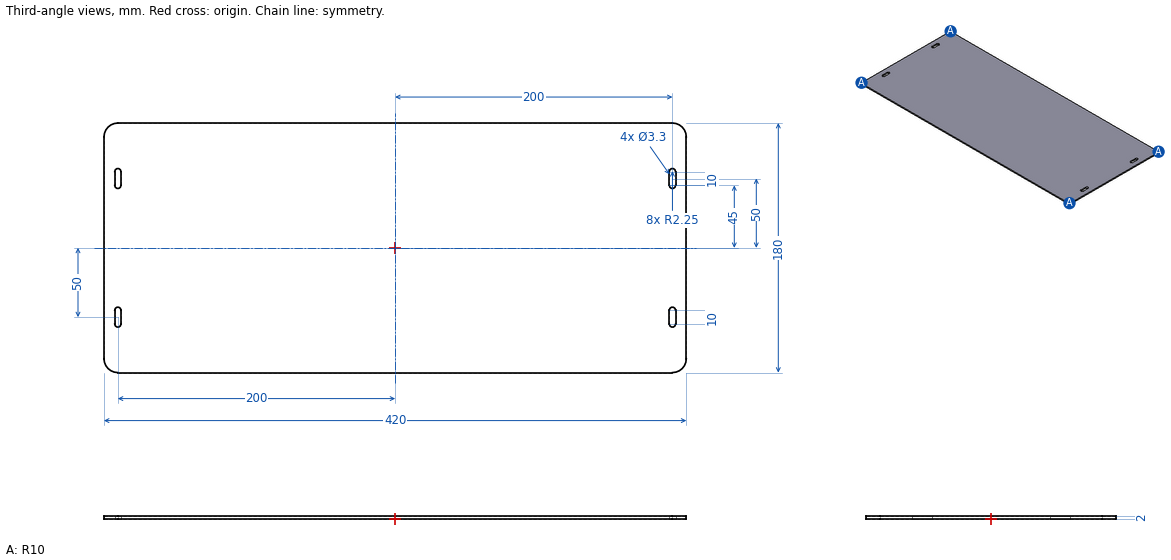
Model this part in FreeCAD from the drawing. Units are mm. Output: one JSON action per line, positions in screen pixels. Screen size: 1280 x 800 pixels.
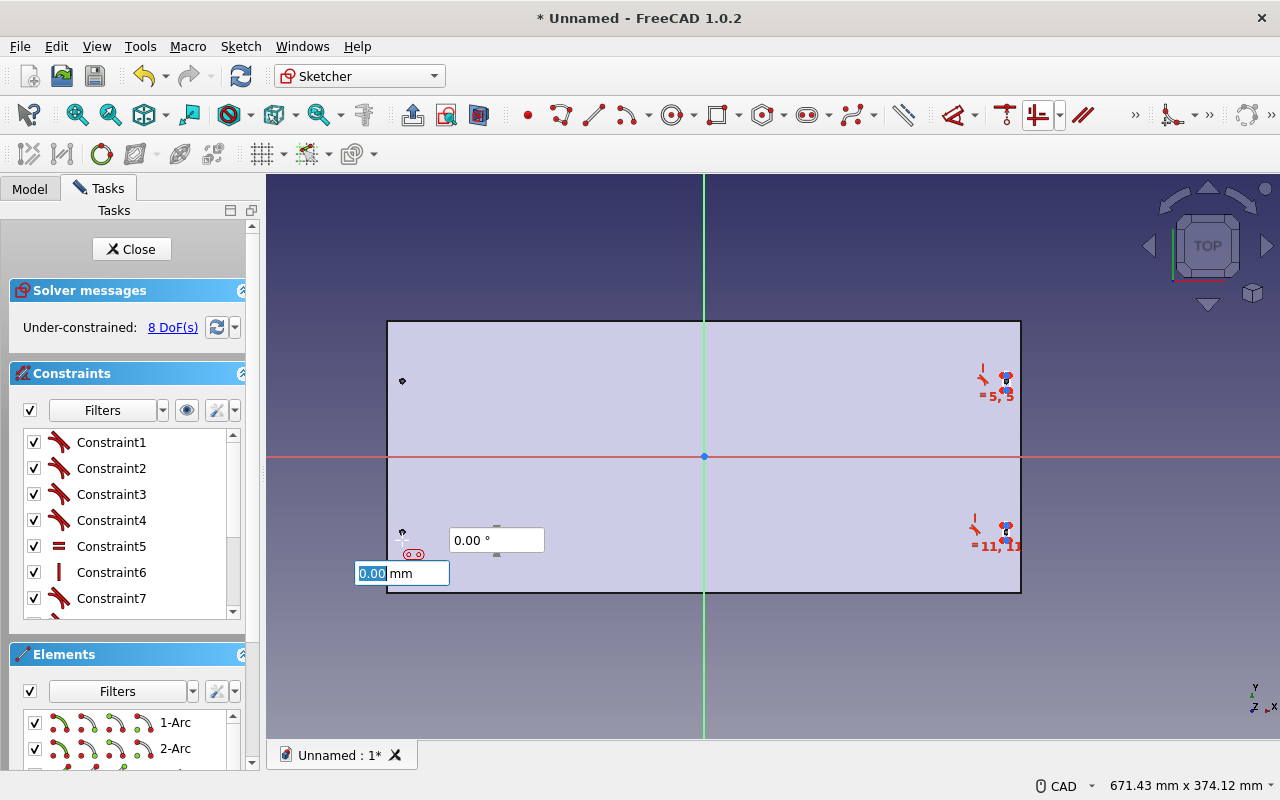
{"action": "left_click", "coordinate": [402, 525]}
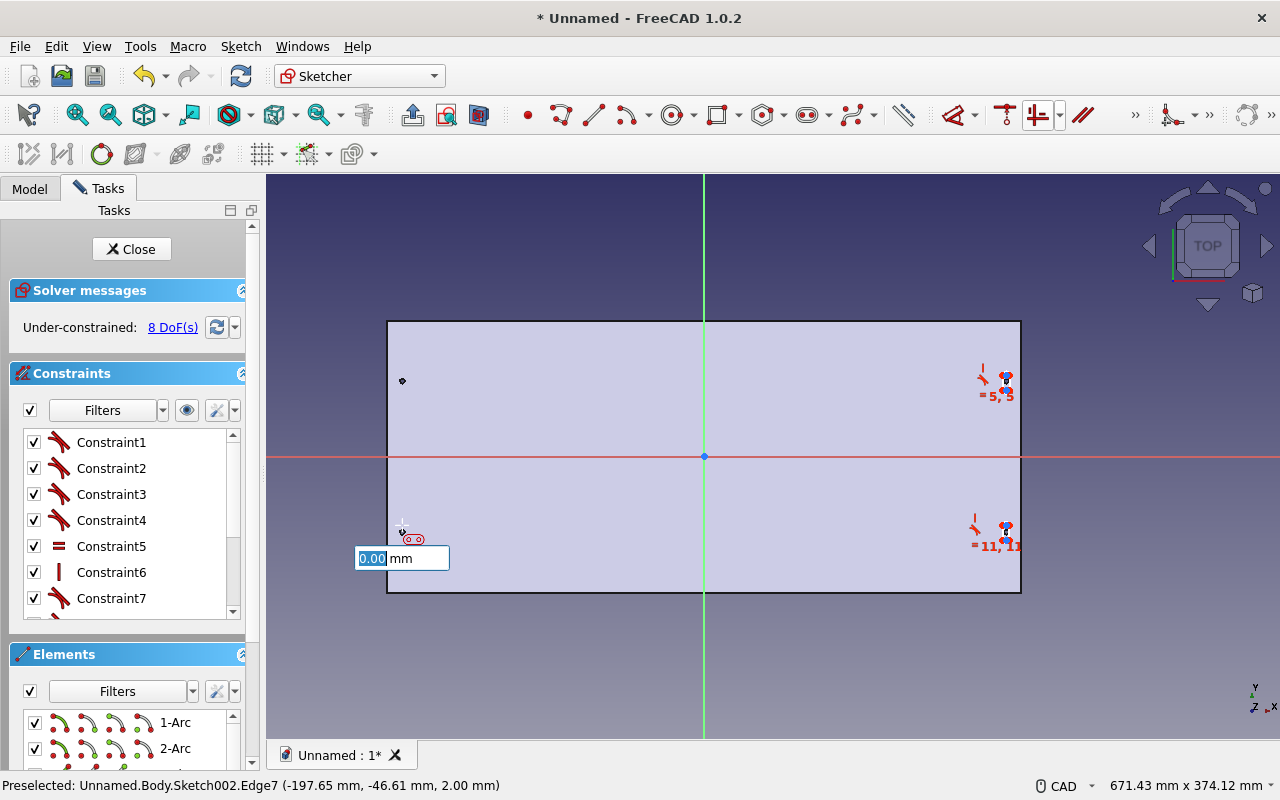
{"action": "scroll", "coordinate": [406, 532], "scroll_direction": "up", "scroll_amount": 8}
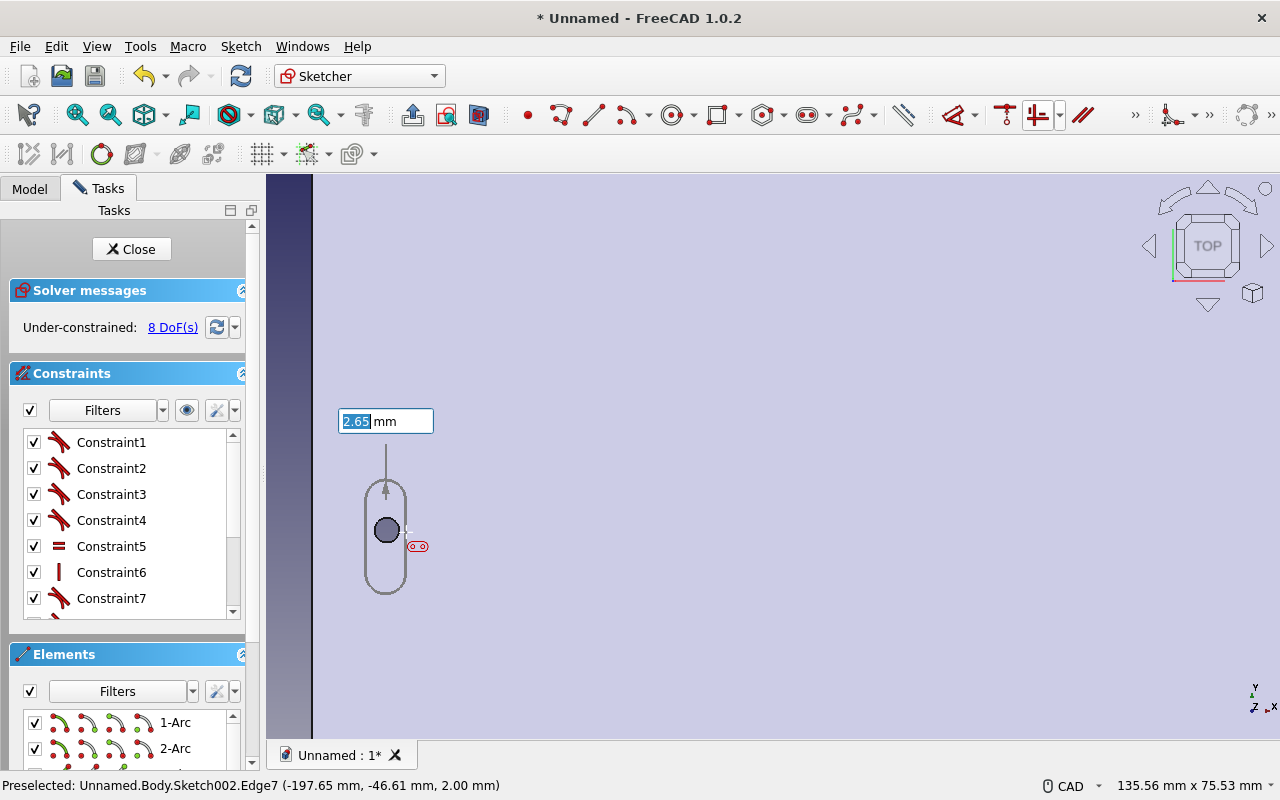
{"action": "left_click", "coordinate": [404, 530]}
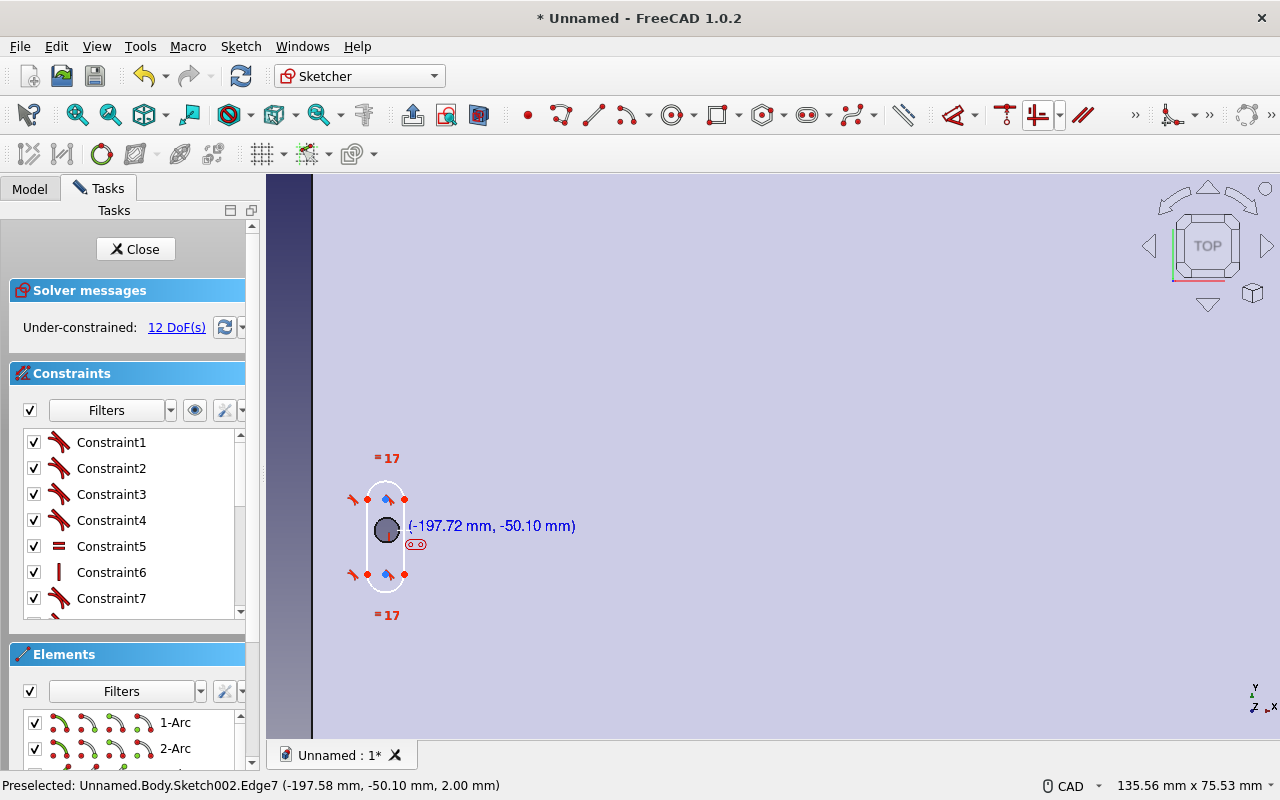
{"action": "scroll", "coordinate": [406, 532], "scroll_direction": "down", "scroll_amount": 8}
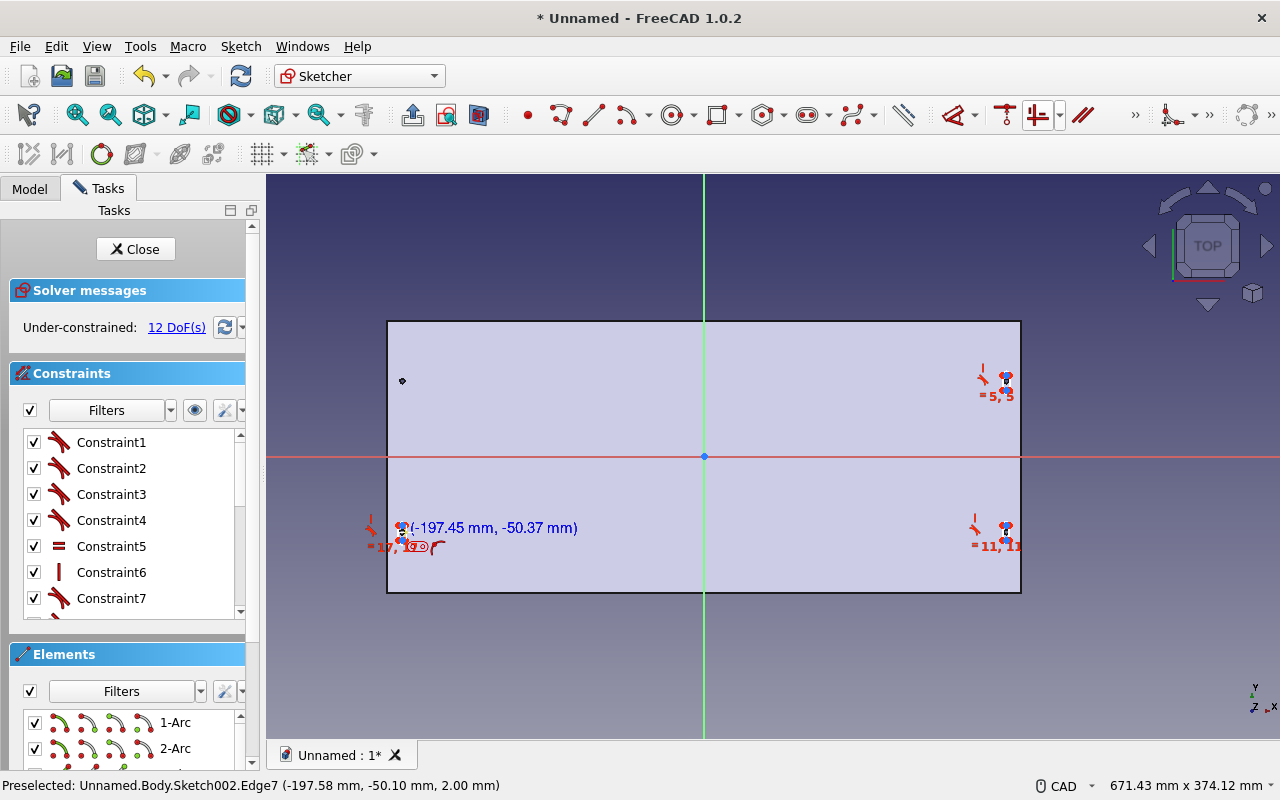
{"action": "scroll", "coordinate": [402, 389], "scroll_direction": "up", "scroll_amount": 10}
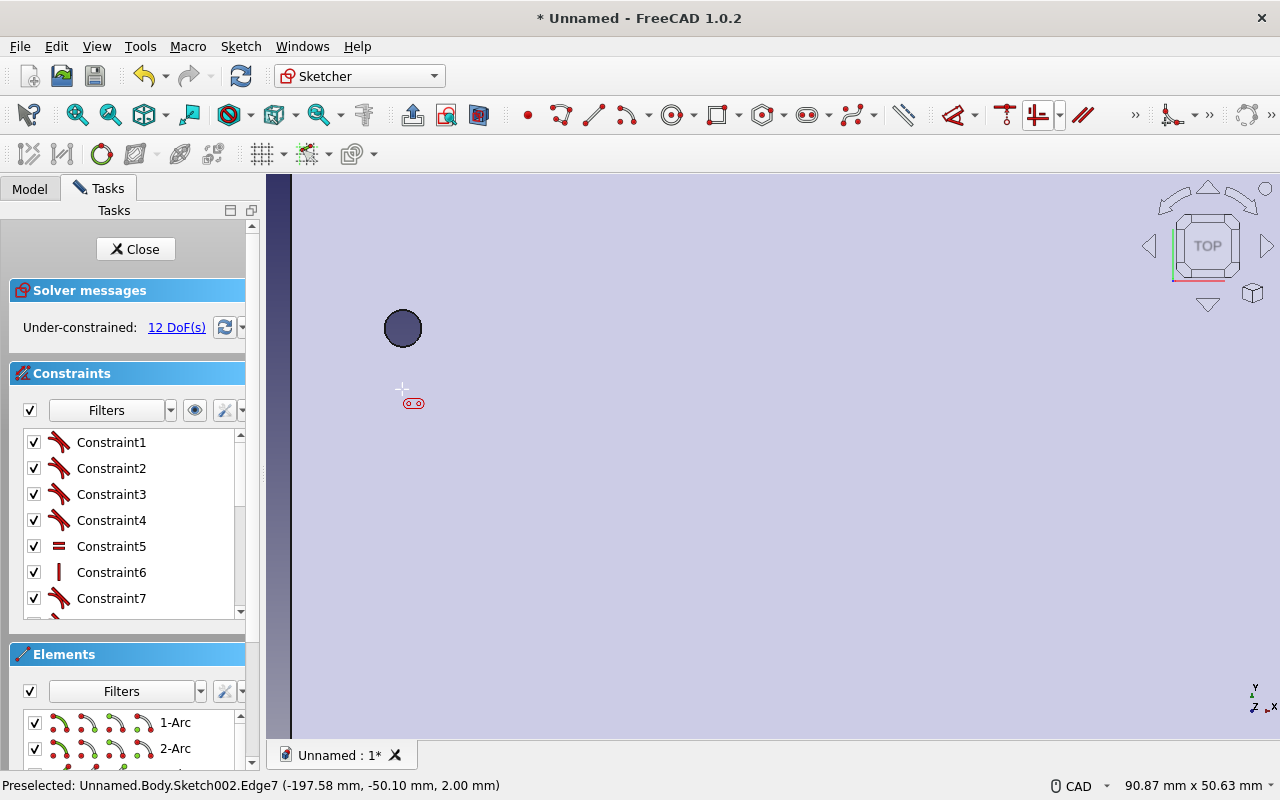
{"action": "scroll", "coordinate": [402, 389], "scroll_direction": "down", "scroll_amount": 10}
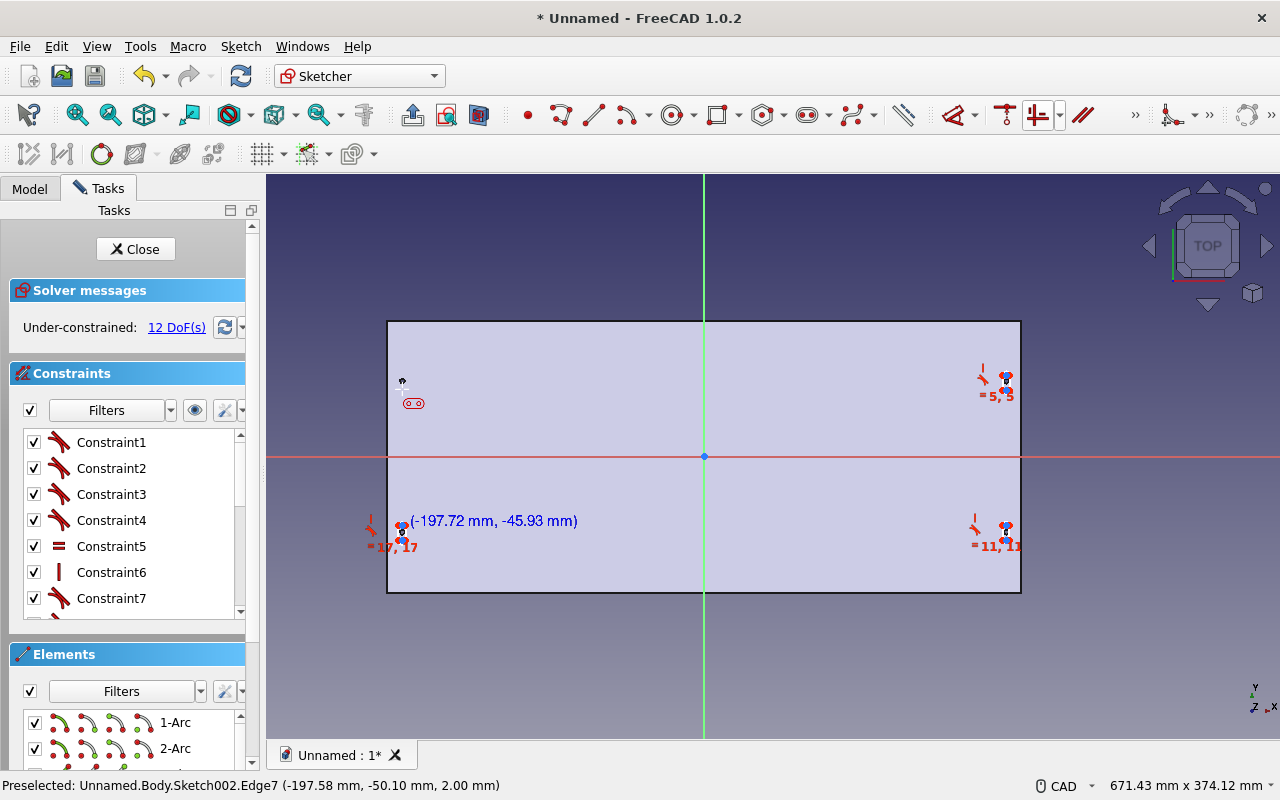
{"action": "left_click", "coordinate": [402, 389]}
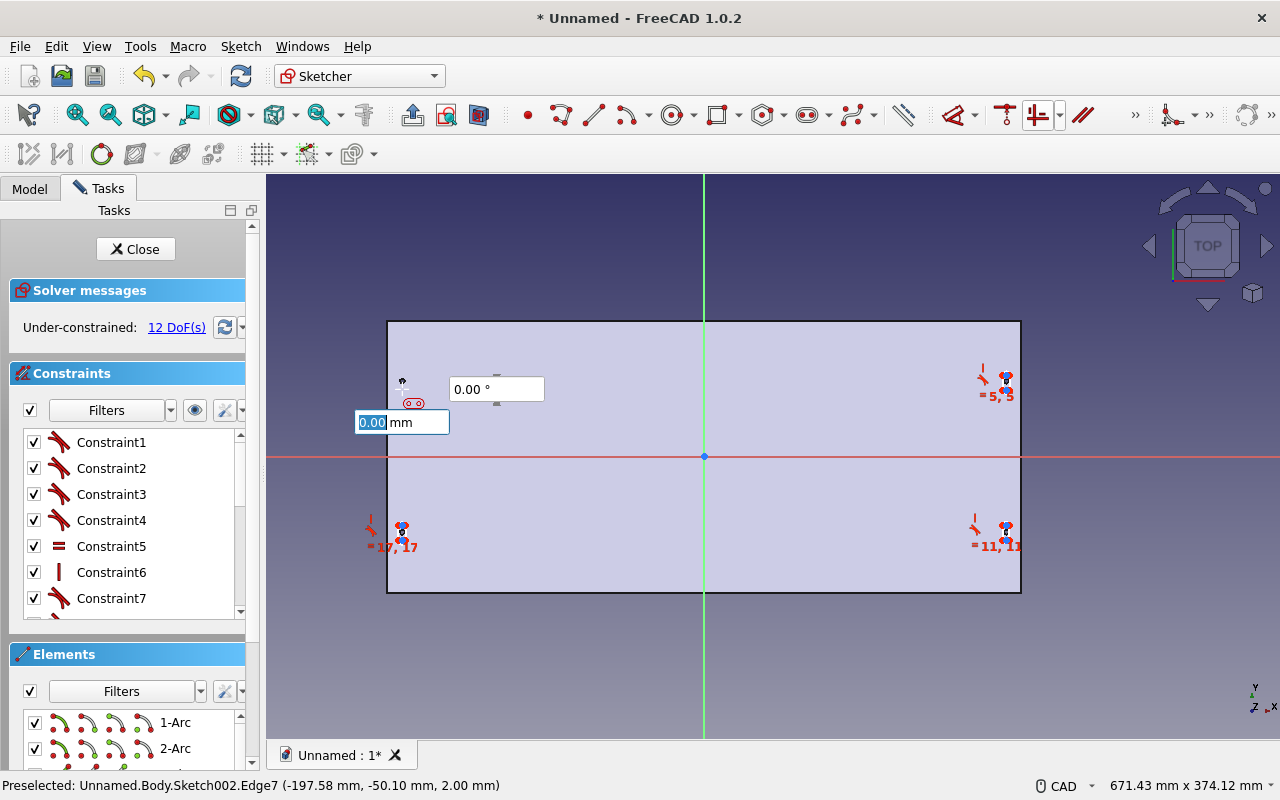
{"action": "left_click", "coordinate": [402, 374]}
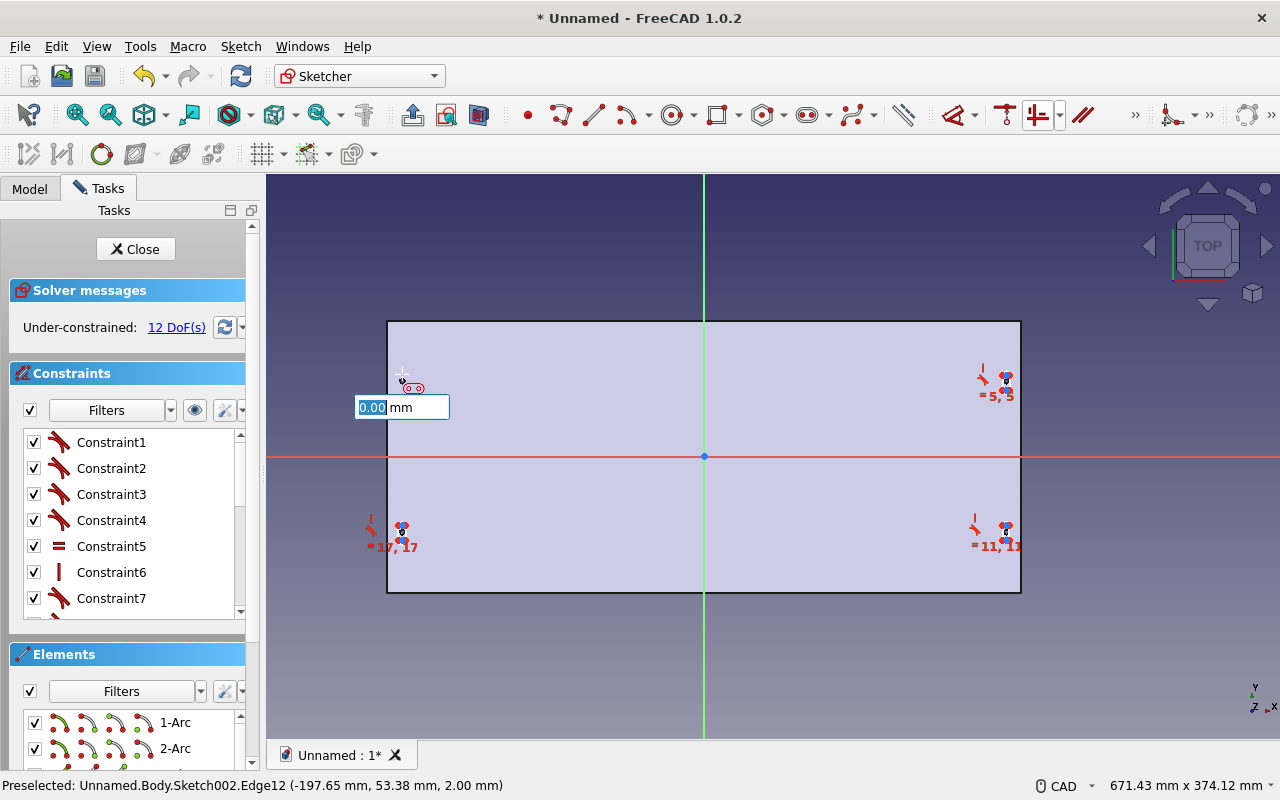
{"action": "scroll", "coordinate": [399, 381], "scroll_direction": "up", "scroll_amount": 8}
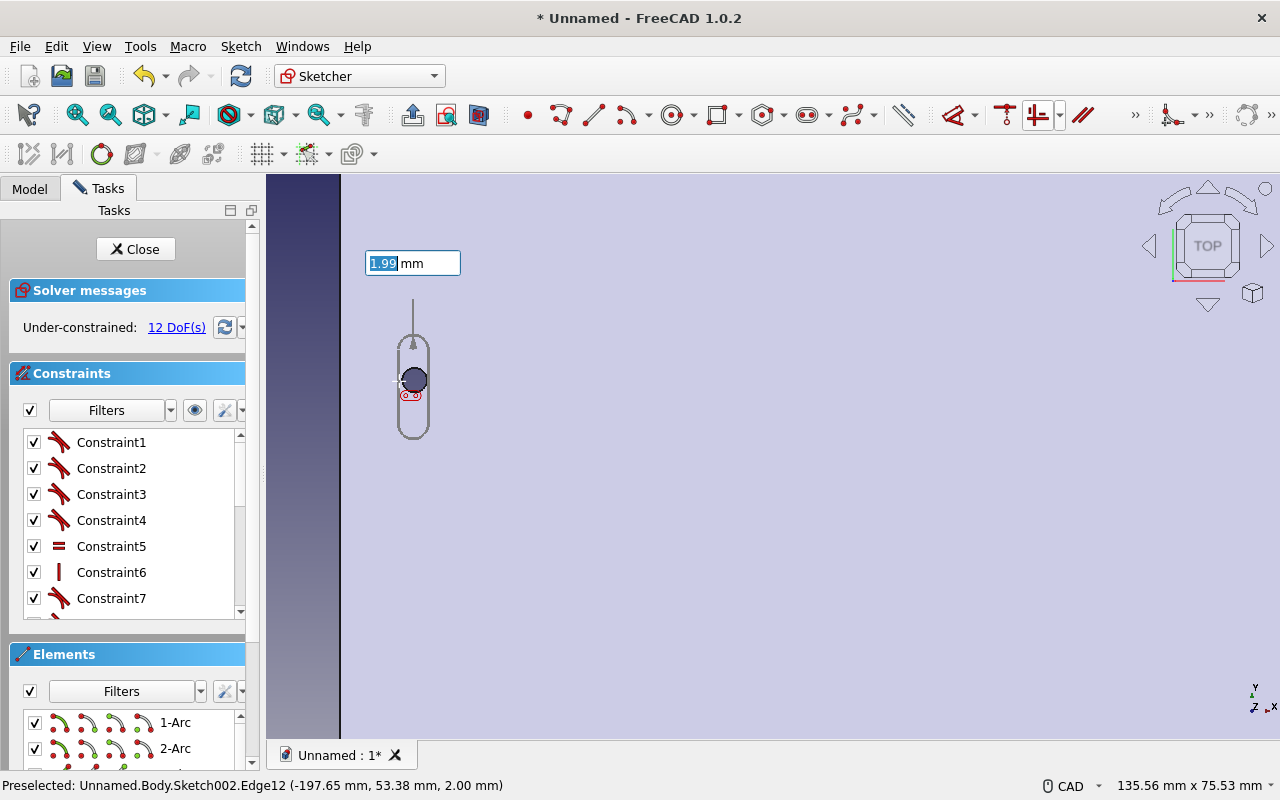
{"action": "left_click", "coordinate": [398, 380]}
{"action": "key", "text": "Escape"}